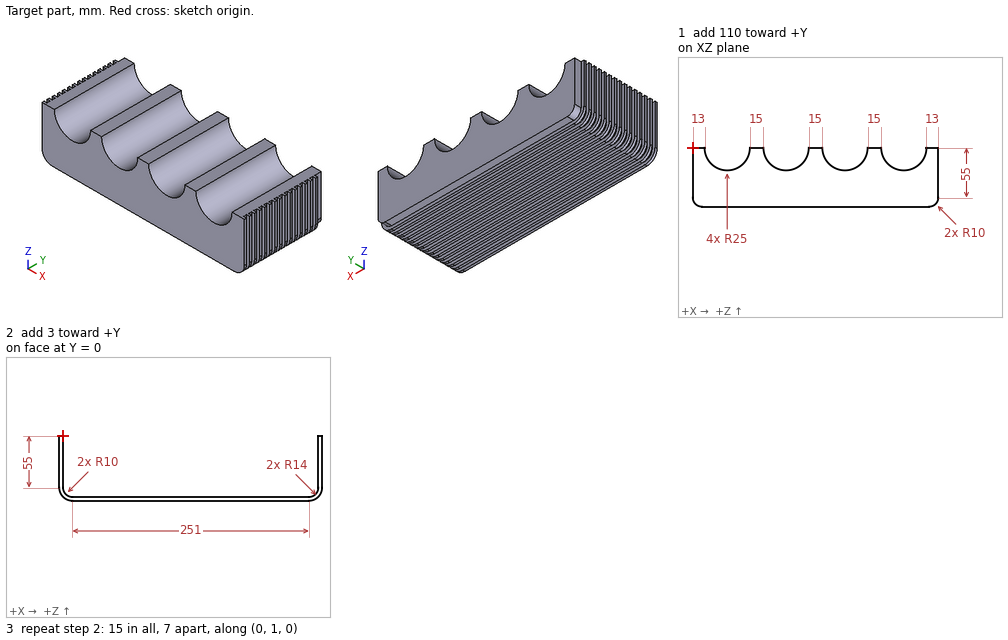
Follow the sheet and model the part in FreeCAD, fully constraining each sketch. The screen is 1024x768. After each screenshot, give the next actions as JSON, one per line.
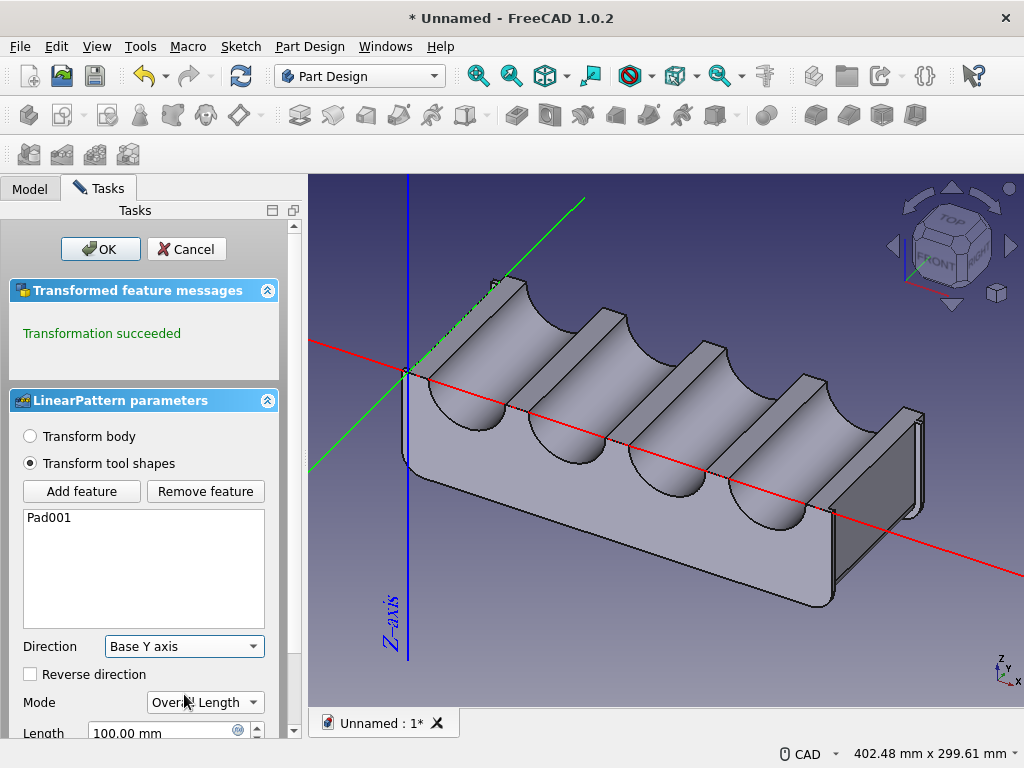
{"action": "left_click", "coordinate": [206, 702]}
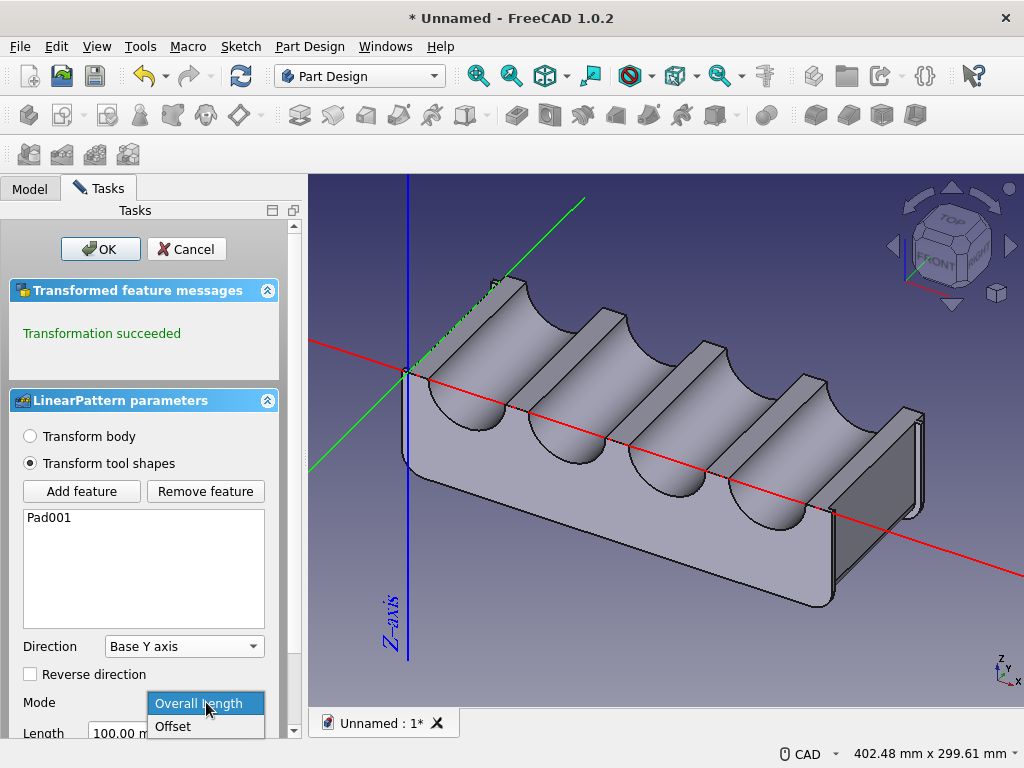
{"action": "left_click", "coordinate": [204, 726]}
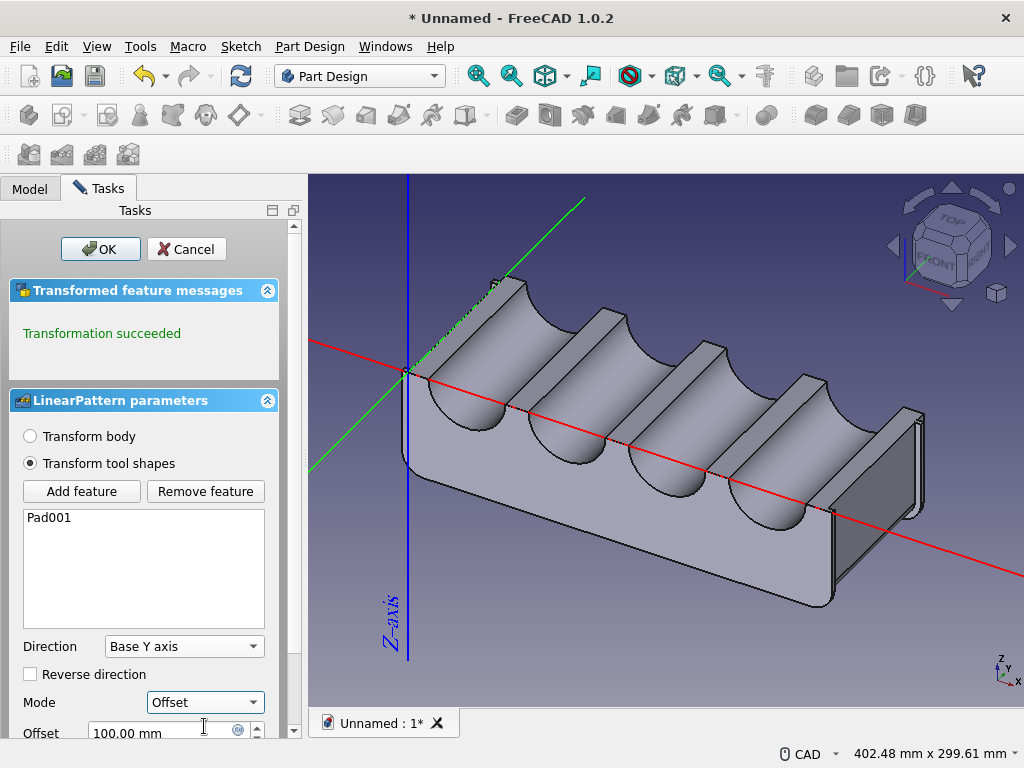
{"action": "scroll", "coordinate": [294, 479], "scroll_direction": "down", "scroll_amount": 2}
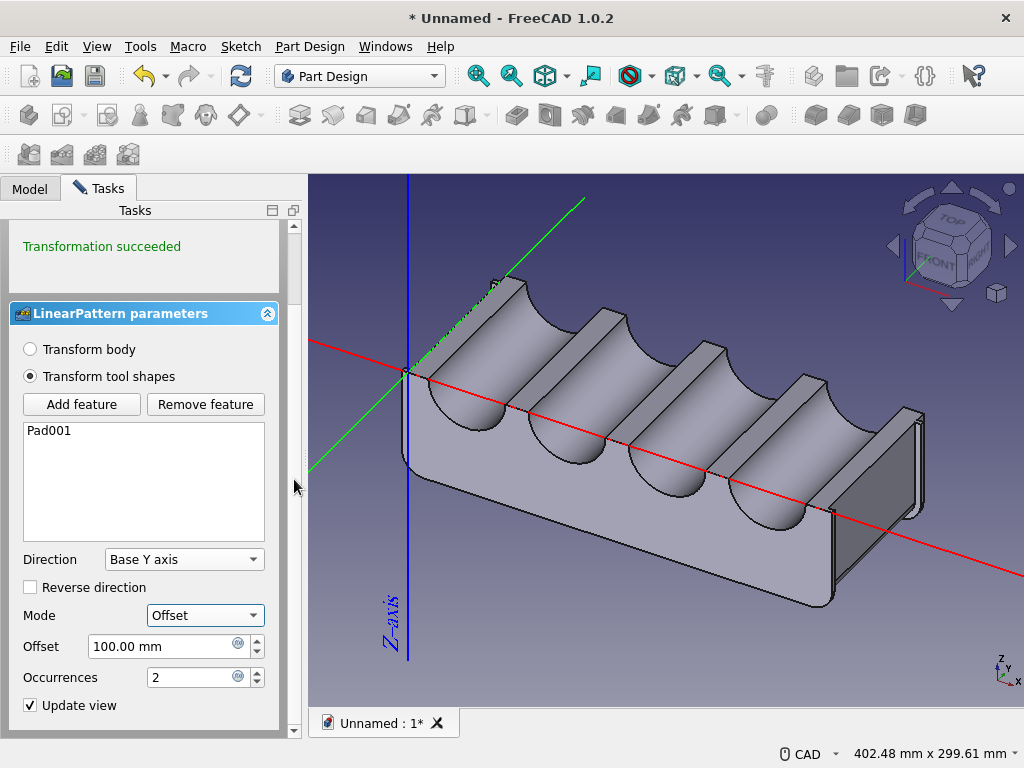
{"action": "triple_click", "coordinate": [170, 646]}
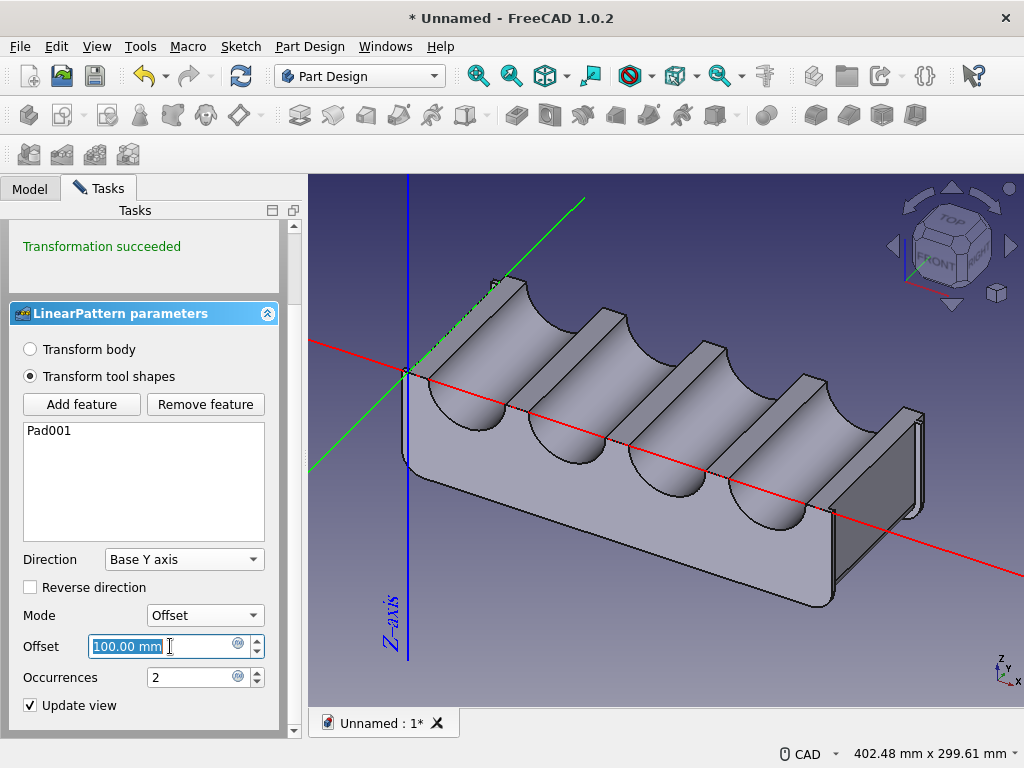
{"action": "type", "text": "7"}
{"action": "key", "text": "Tab"}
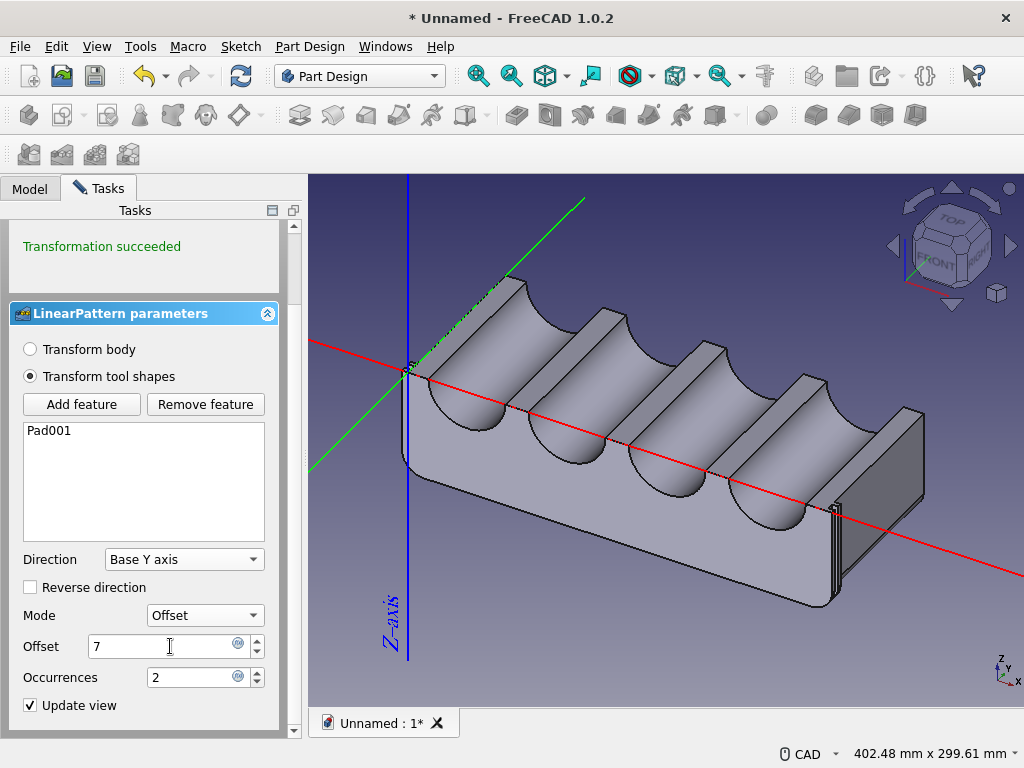
{"action": "triple_click", "coordinate": [199, 678]}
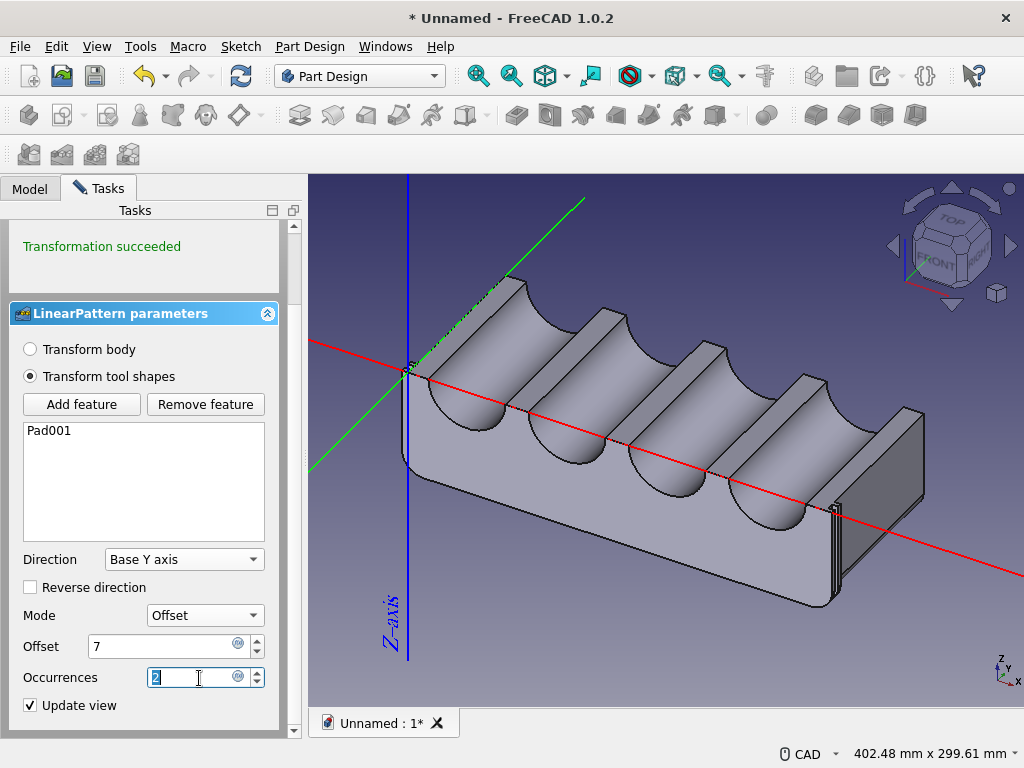
{"action": "type", "text": "15"}
{"action": "key", "text": "Tab"}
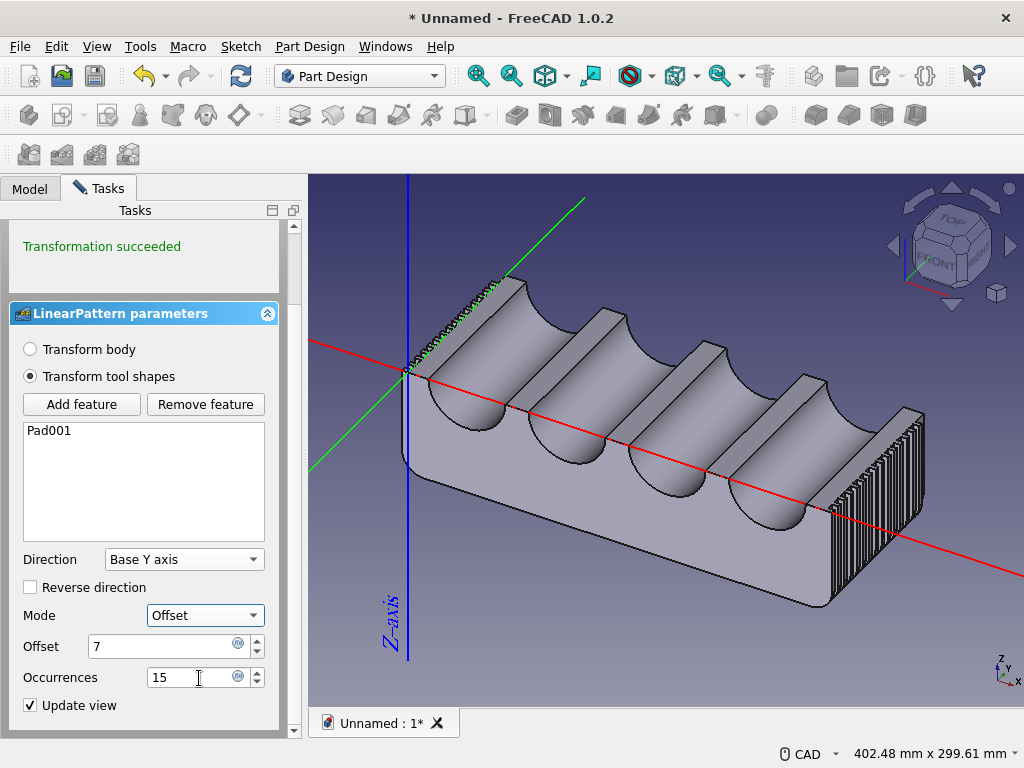
{"action": "scroll", "coordinate": [294, 479], "scroll_direction": "up", "scroll_amount": 3}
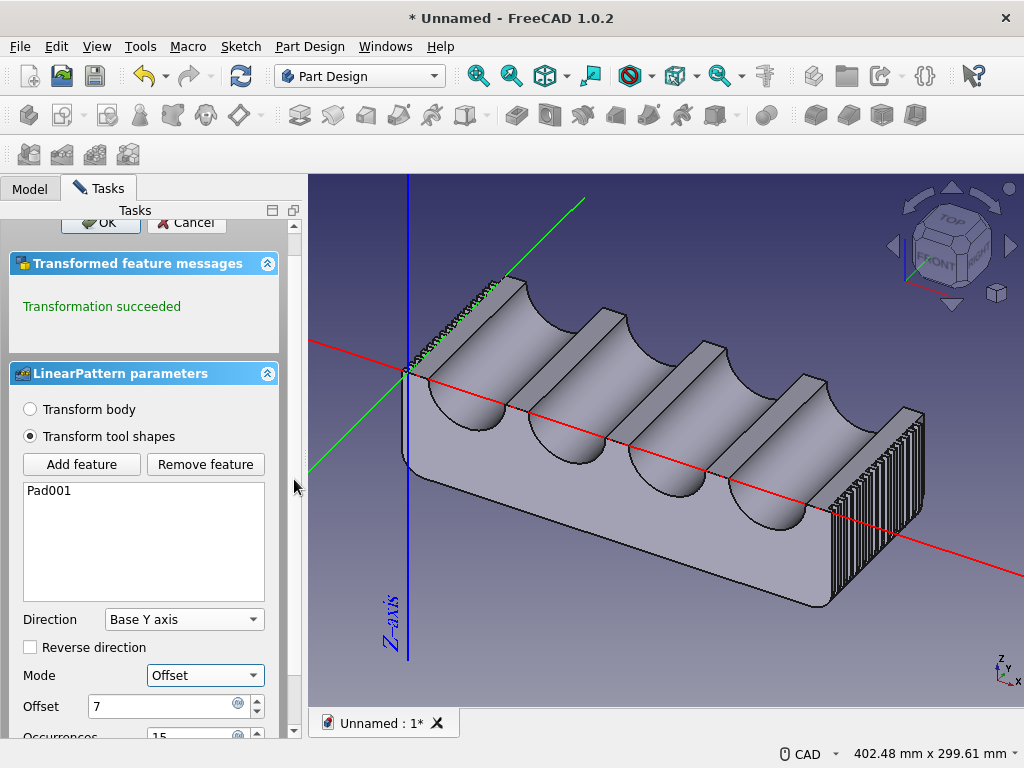
{"action": "left_click", "coordinate": [101, 249]}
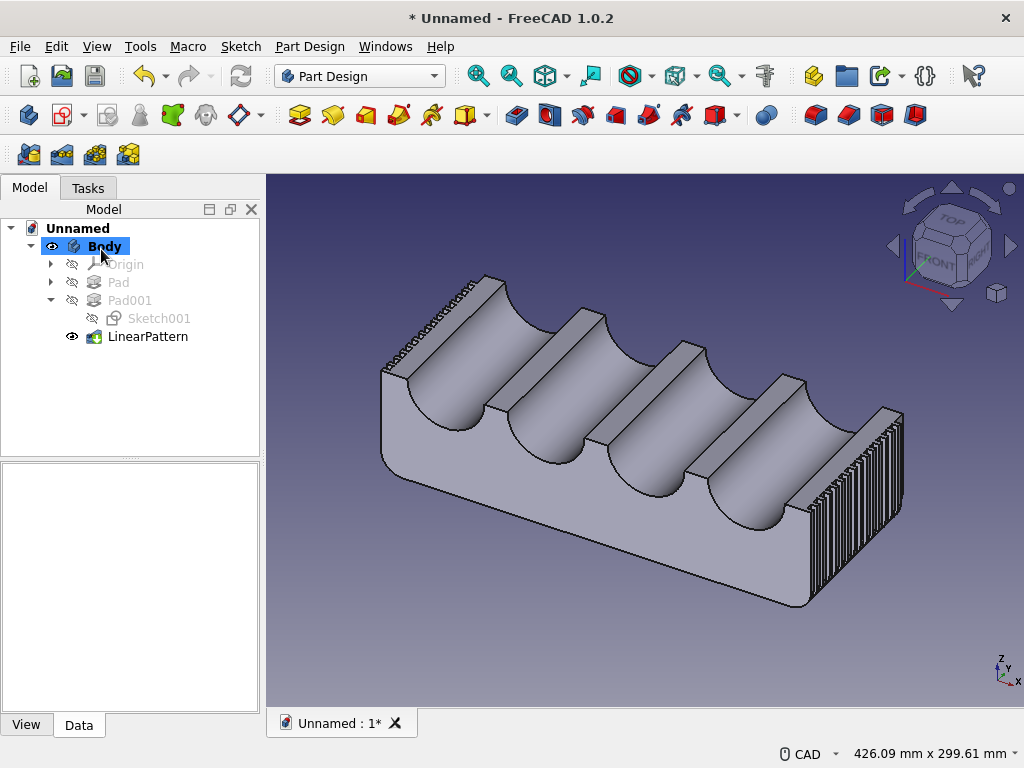
{"action": "key", "text": "0"}